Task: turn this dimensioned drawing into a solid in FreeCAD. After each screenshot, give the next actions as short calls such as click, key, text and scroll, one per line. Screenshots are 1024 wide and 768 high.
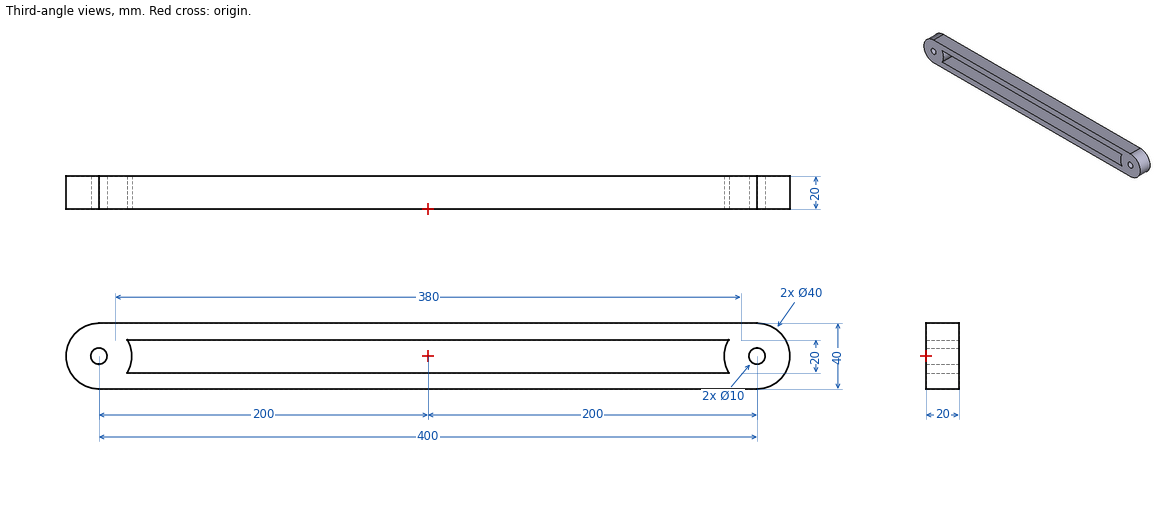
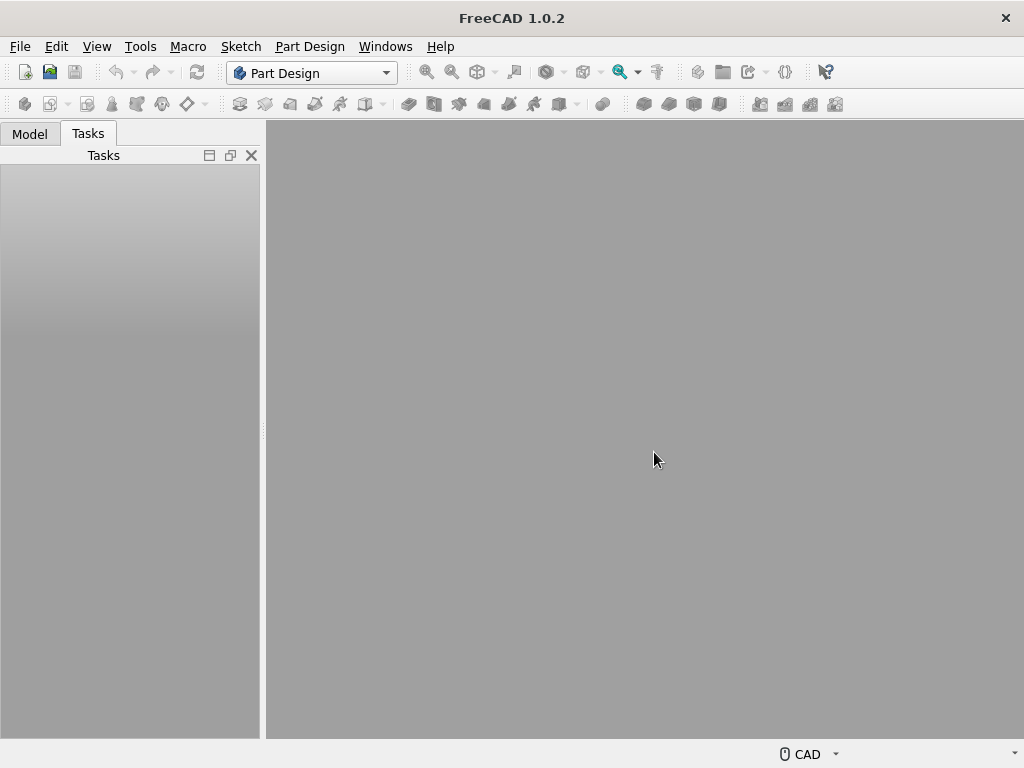
click(25, 72)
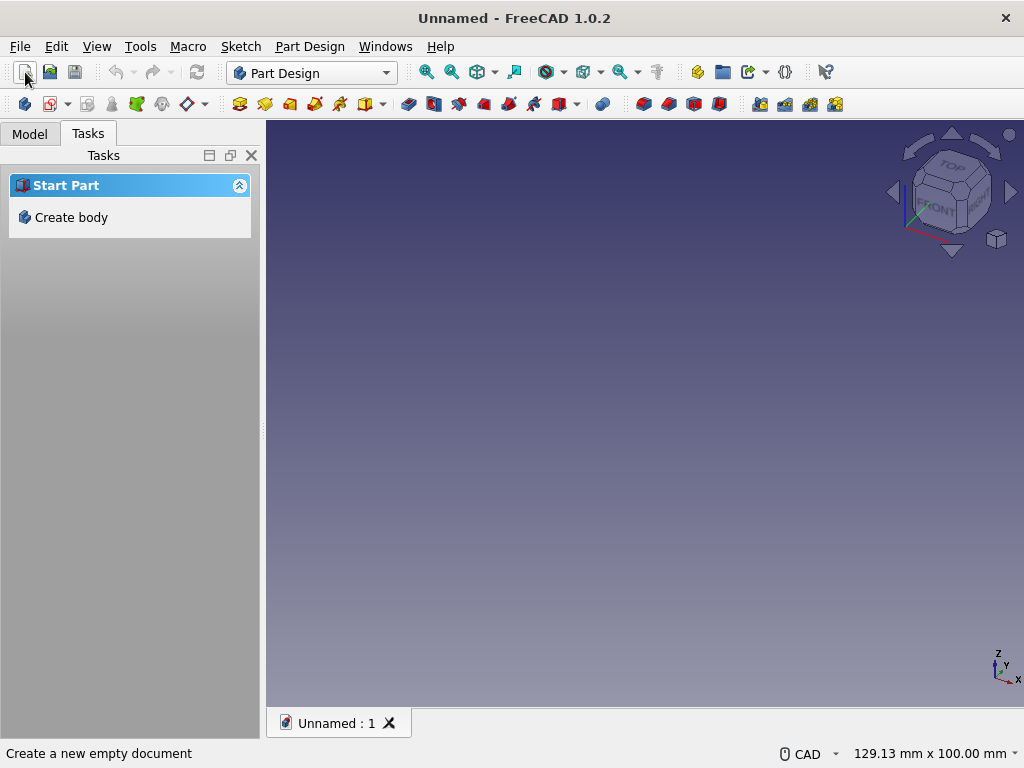
click(50, 104)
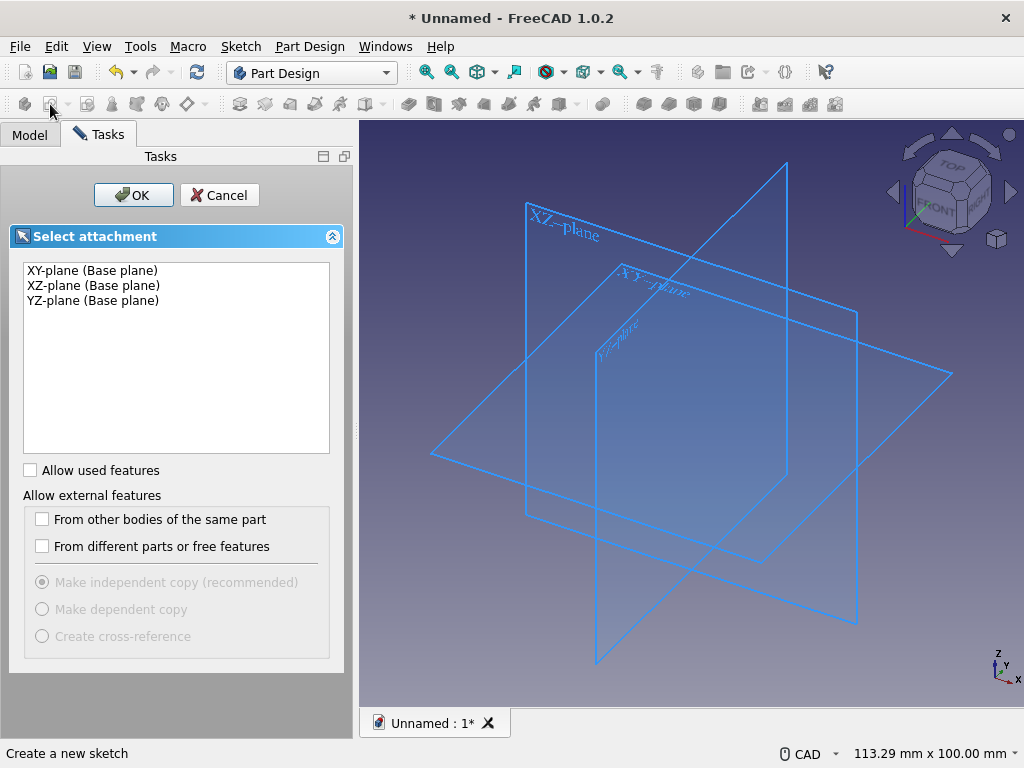
click(84, 286)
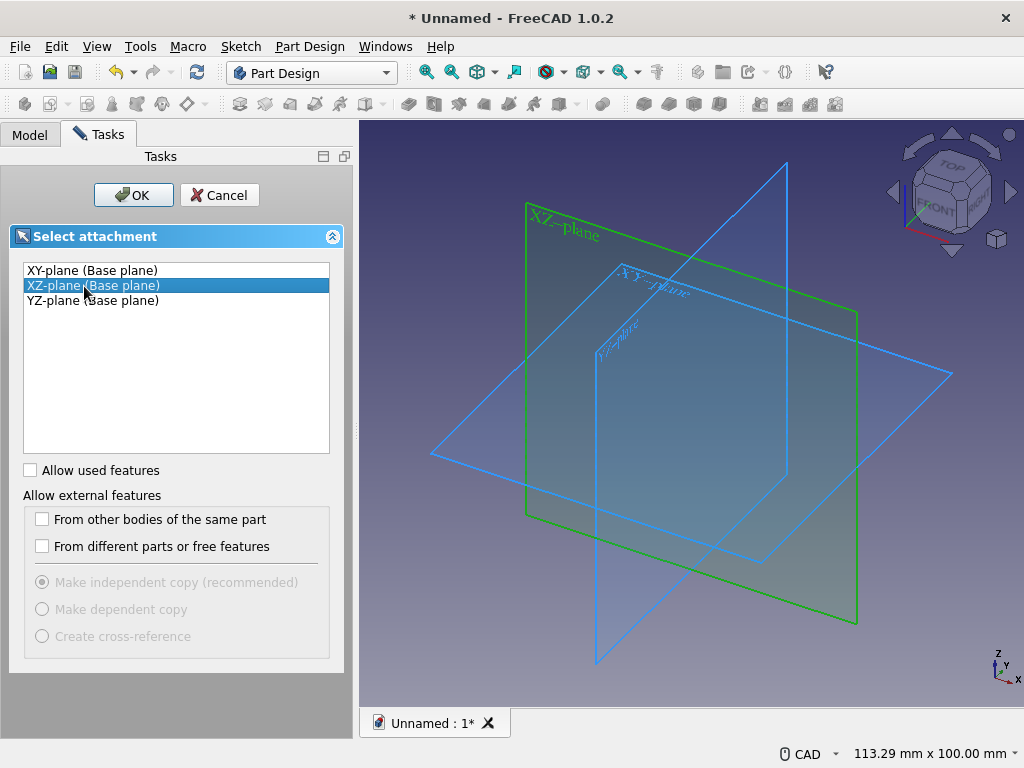
click(134, 195)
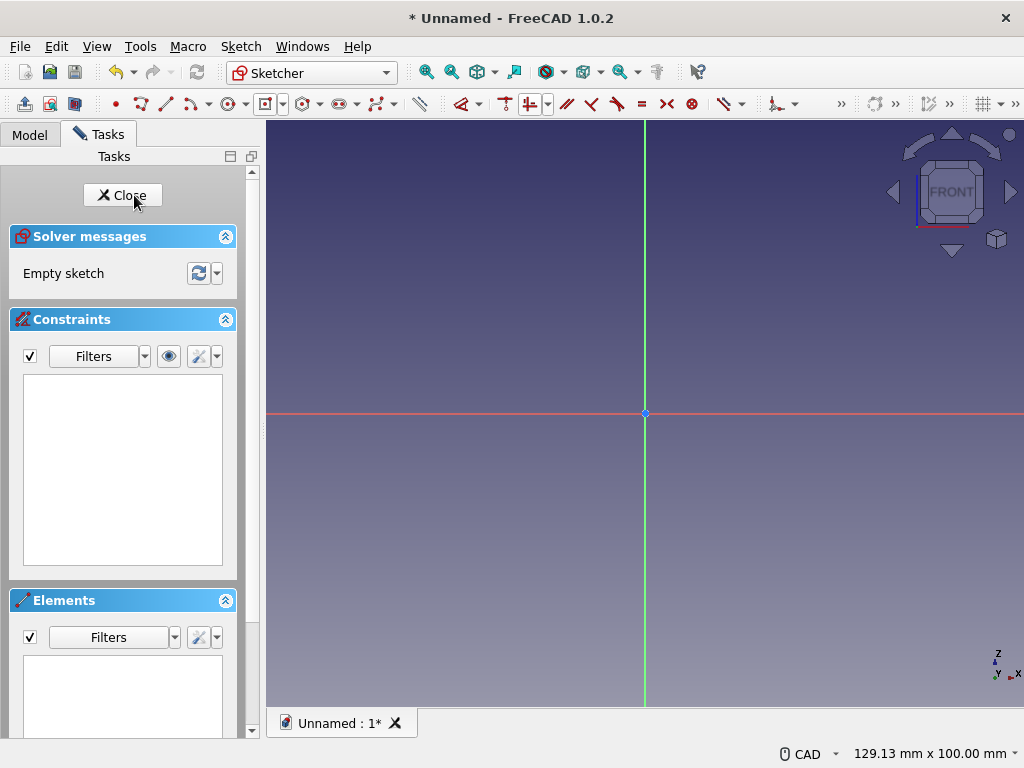
scroll(563, 414, down, 9)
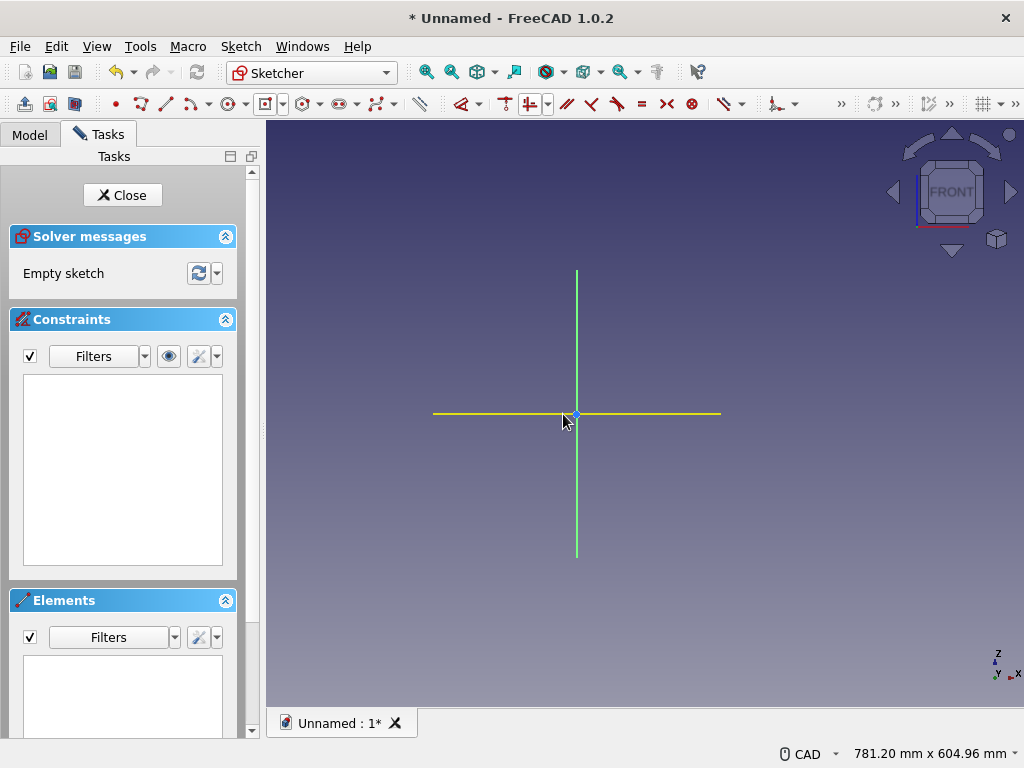
click(264, 104)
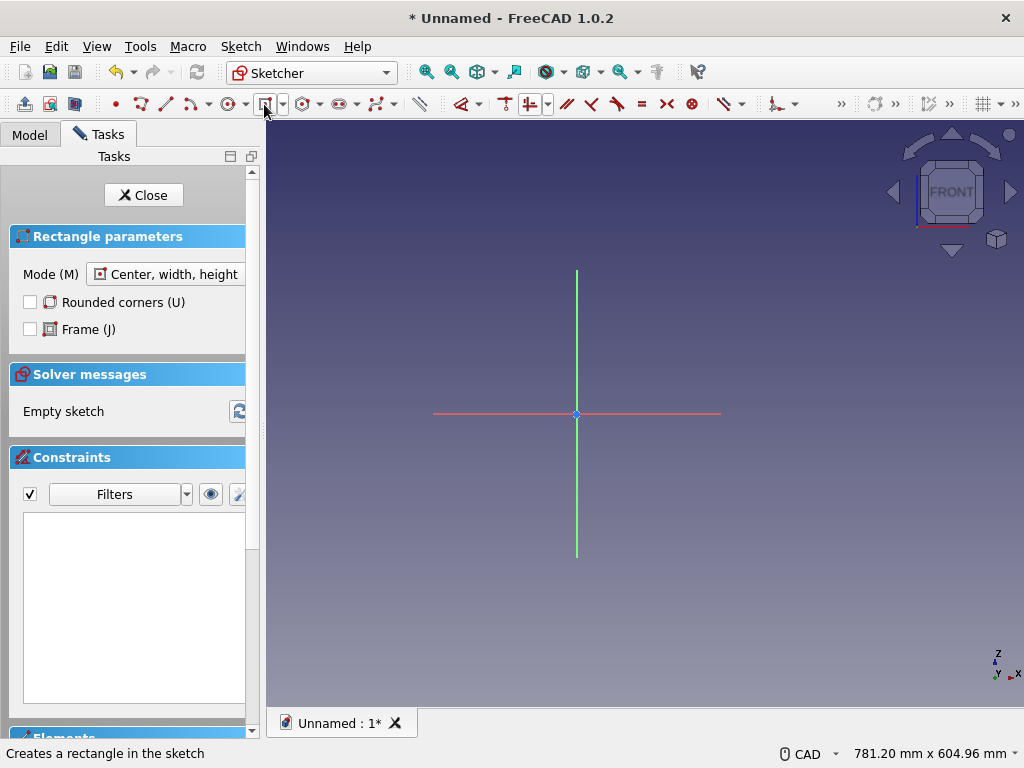
click(577, 414)
click(771, 395)
key(Escape)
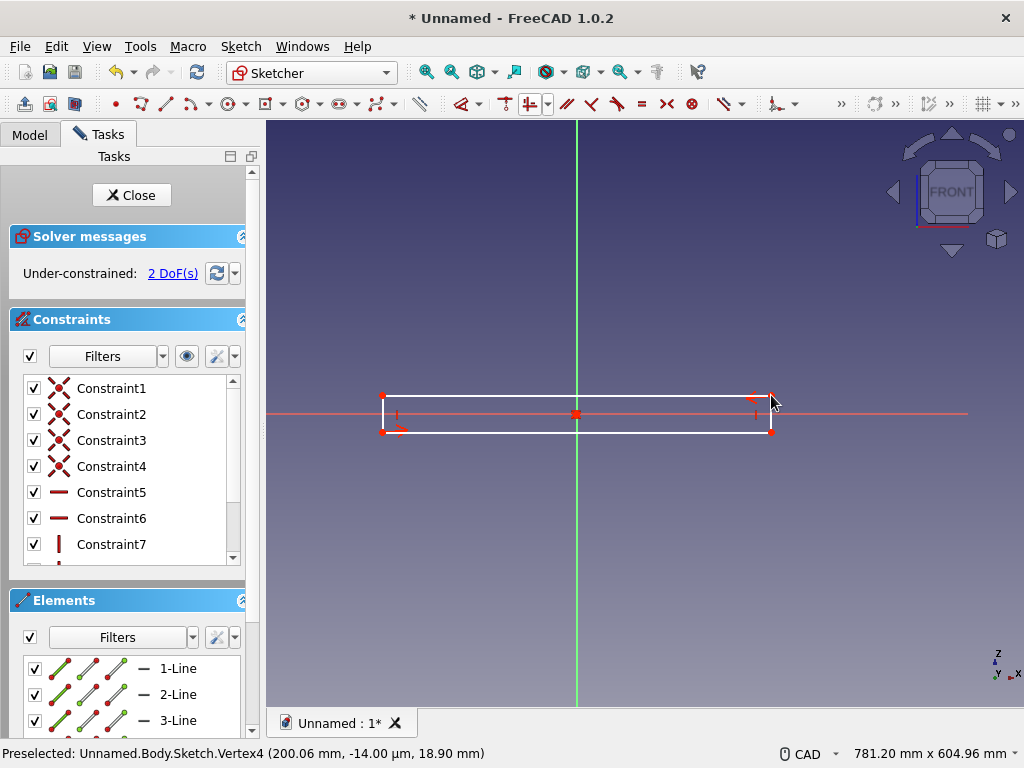
click(460, 104)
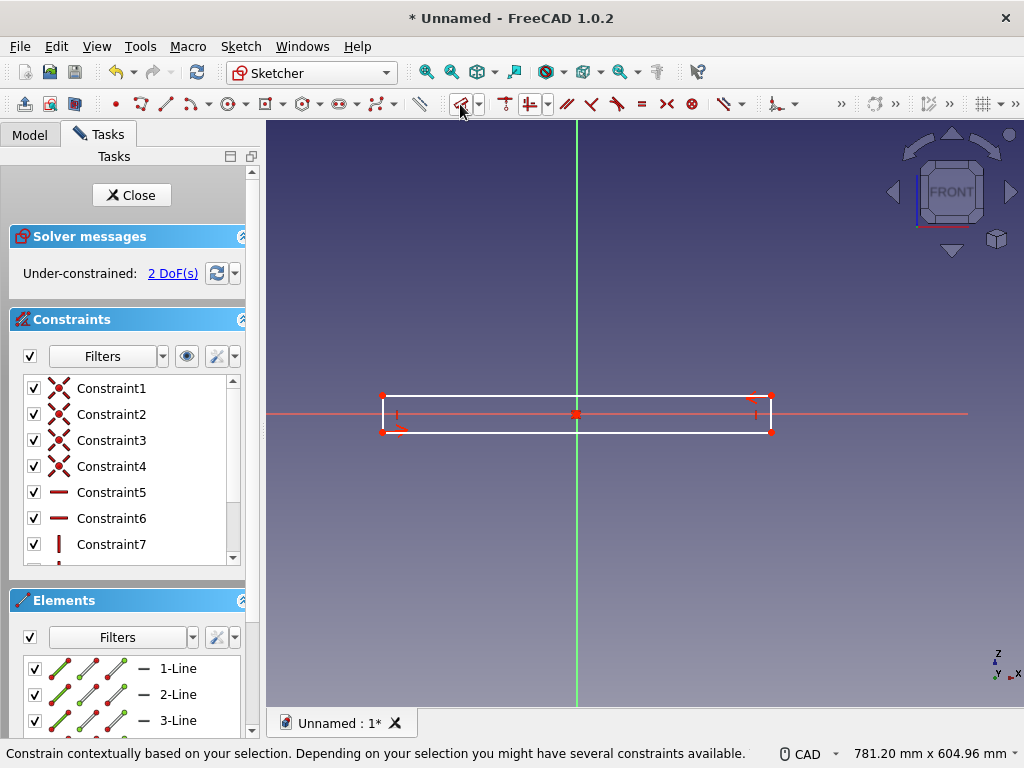
click(771, 418)
click(805, 406)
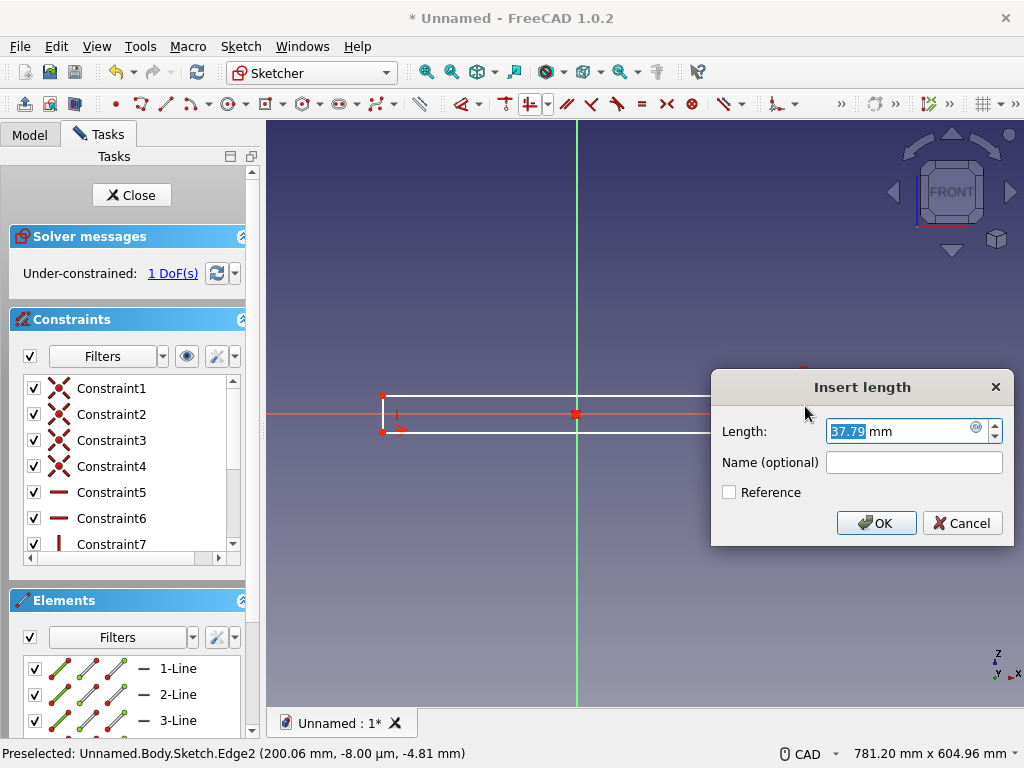
text(40)
key(Return)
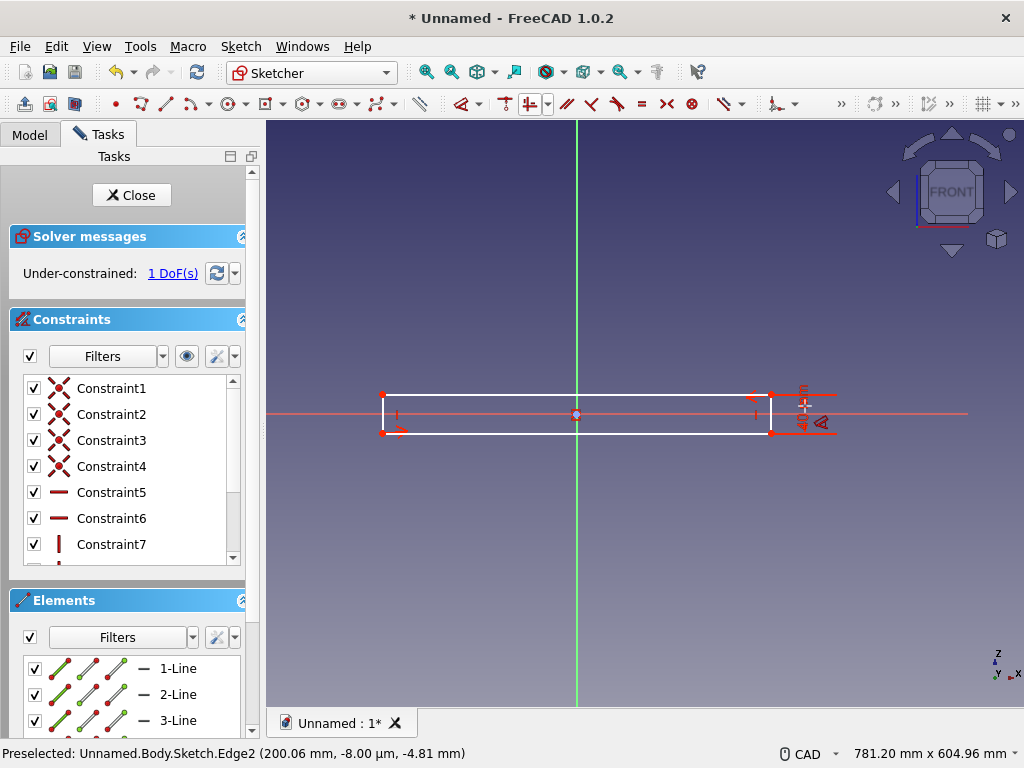
click(499, 434)
click(488, 468)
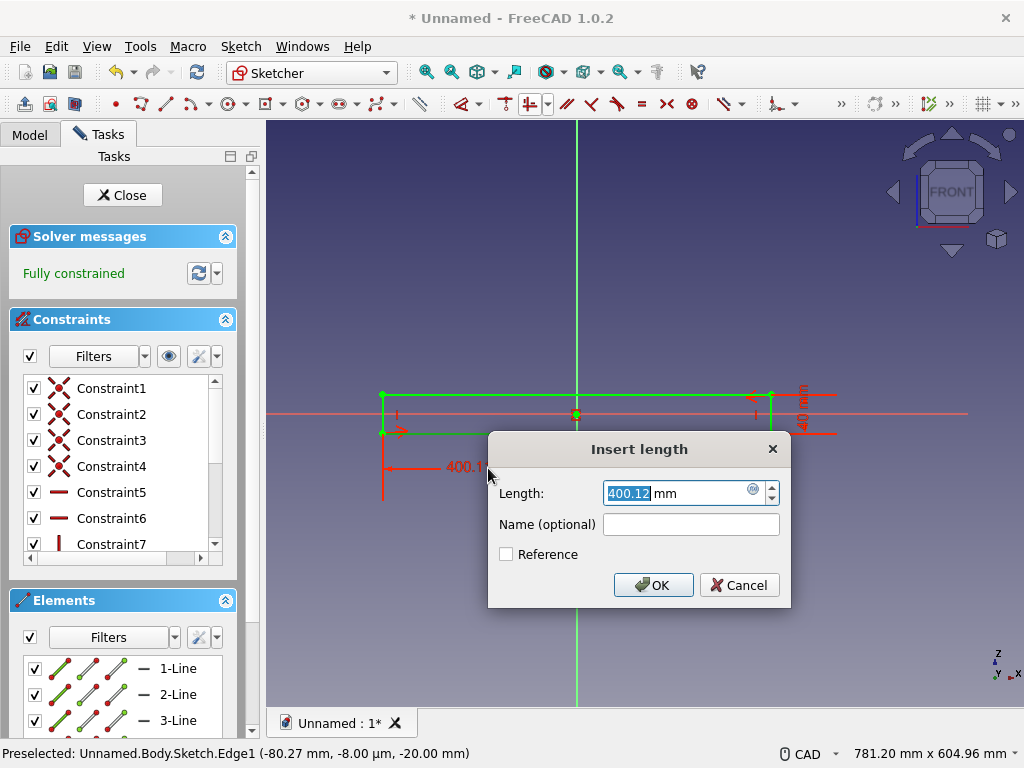
text(400)
key(Return)
key(Escape)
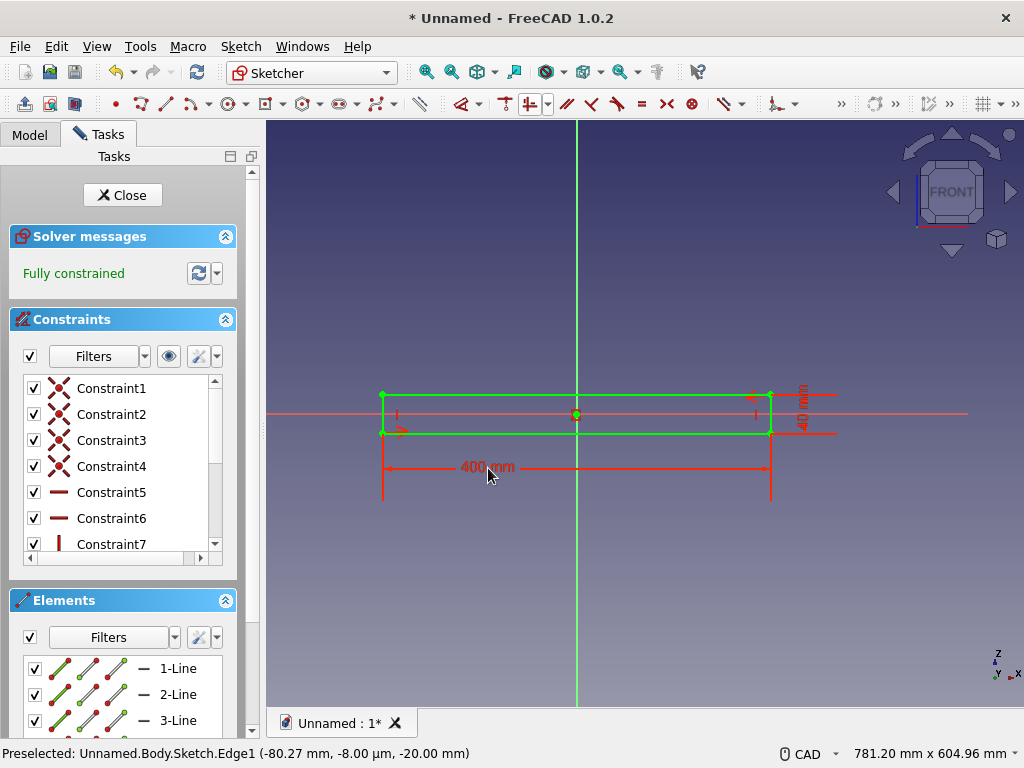
click(123, 195)